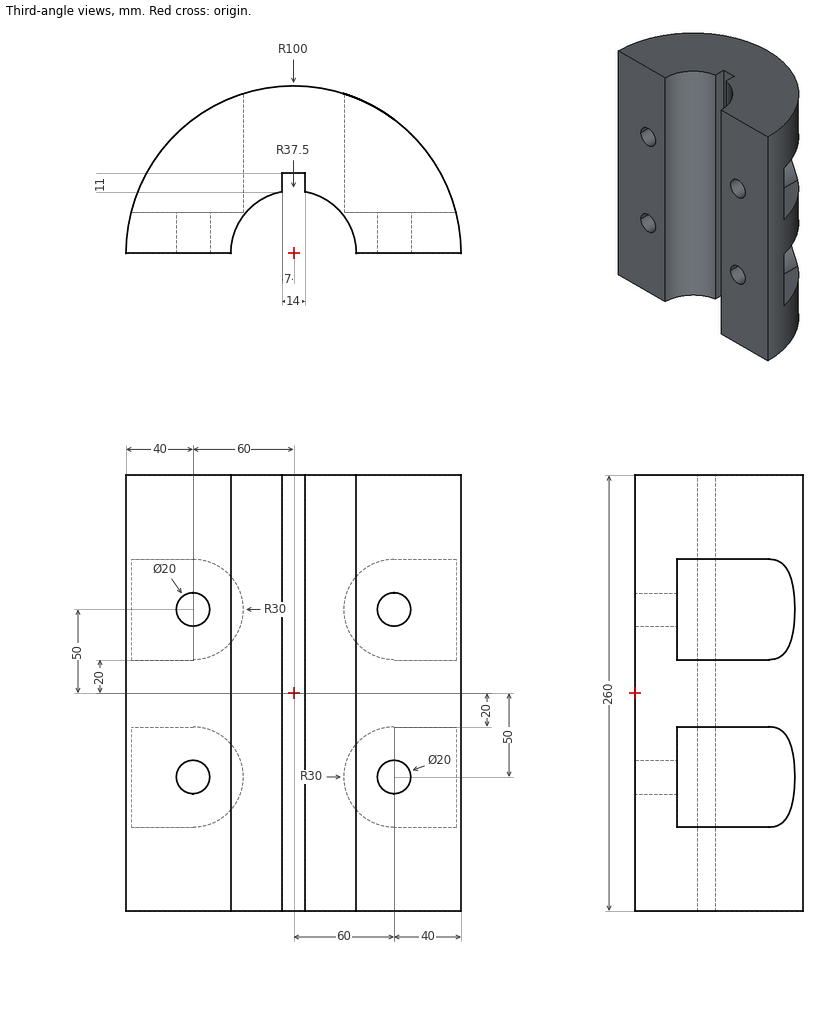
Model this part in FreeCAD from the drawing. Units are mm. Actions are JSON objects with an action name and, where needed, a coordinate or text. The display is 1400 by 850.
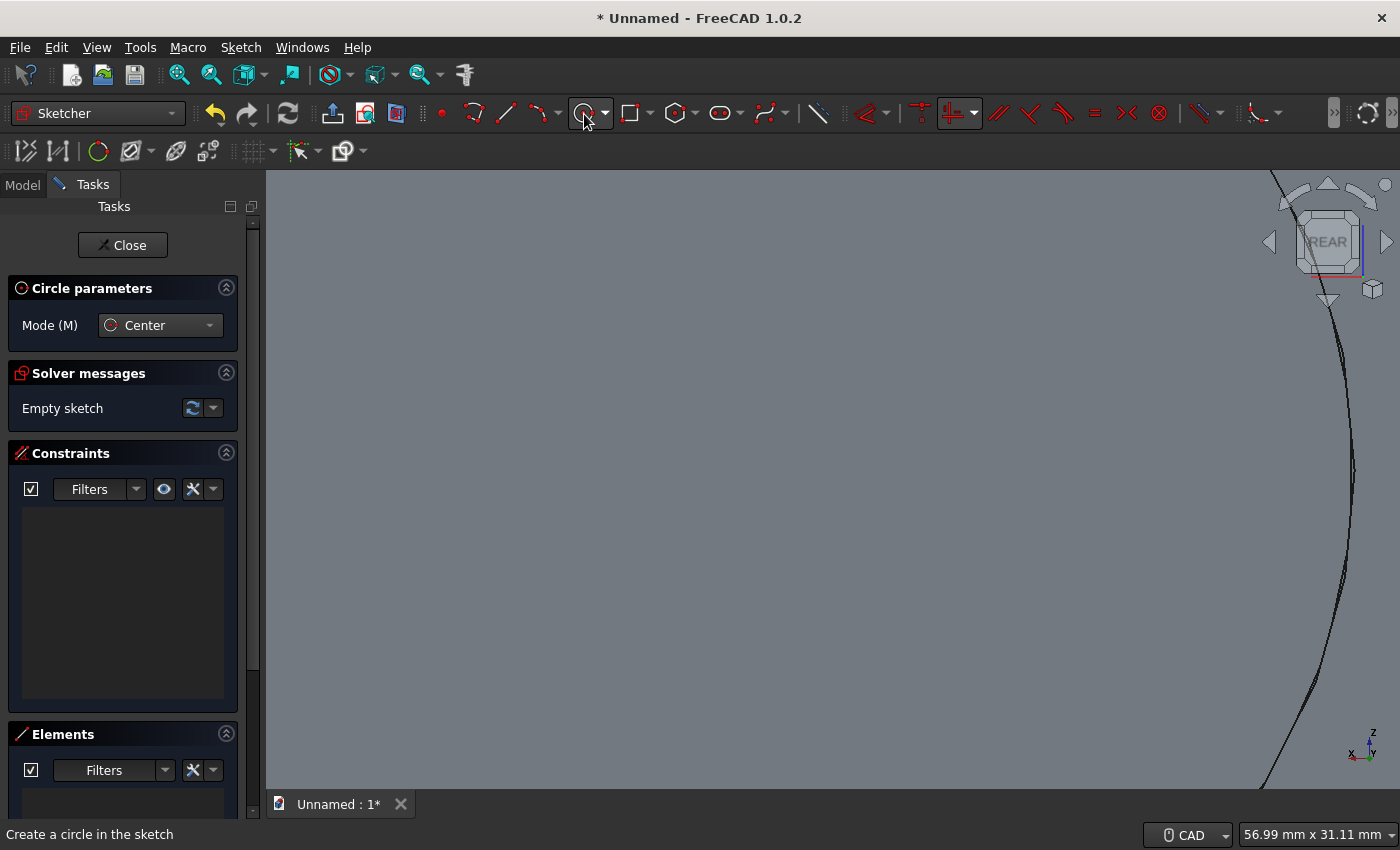
{"action": "left_click", "coordinate": [758, 470]}
{"action": "left_click", "coordinate": [898, 330]}
{"action": "key", "text": "Escape"}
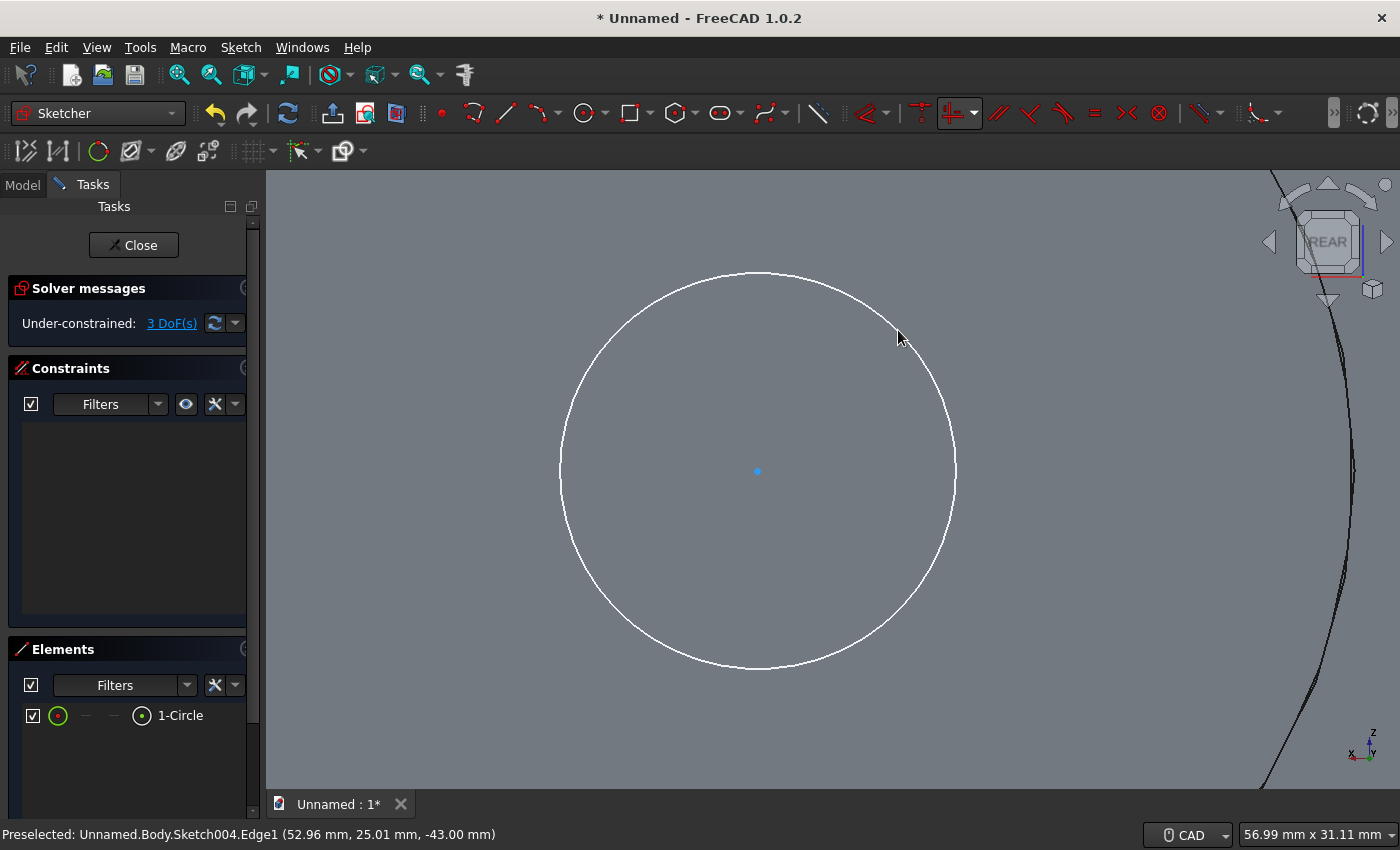
{"action": "left_click", "coordinate": [866, 114]}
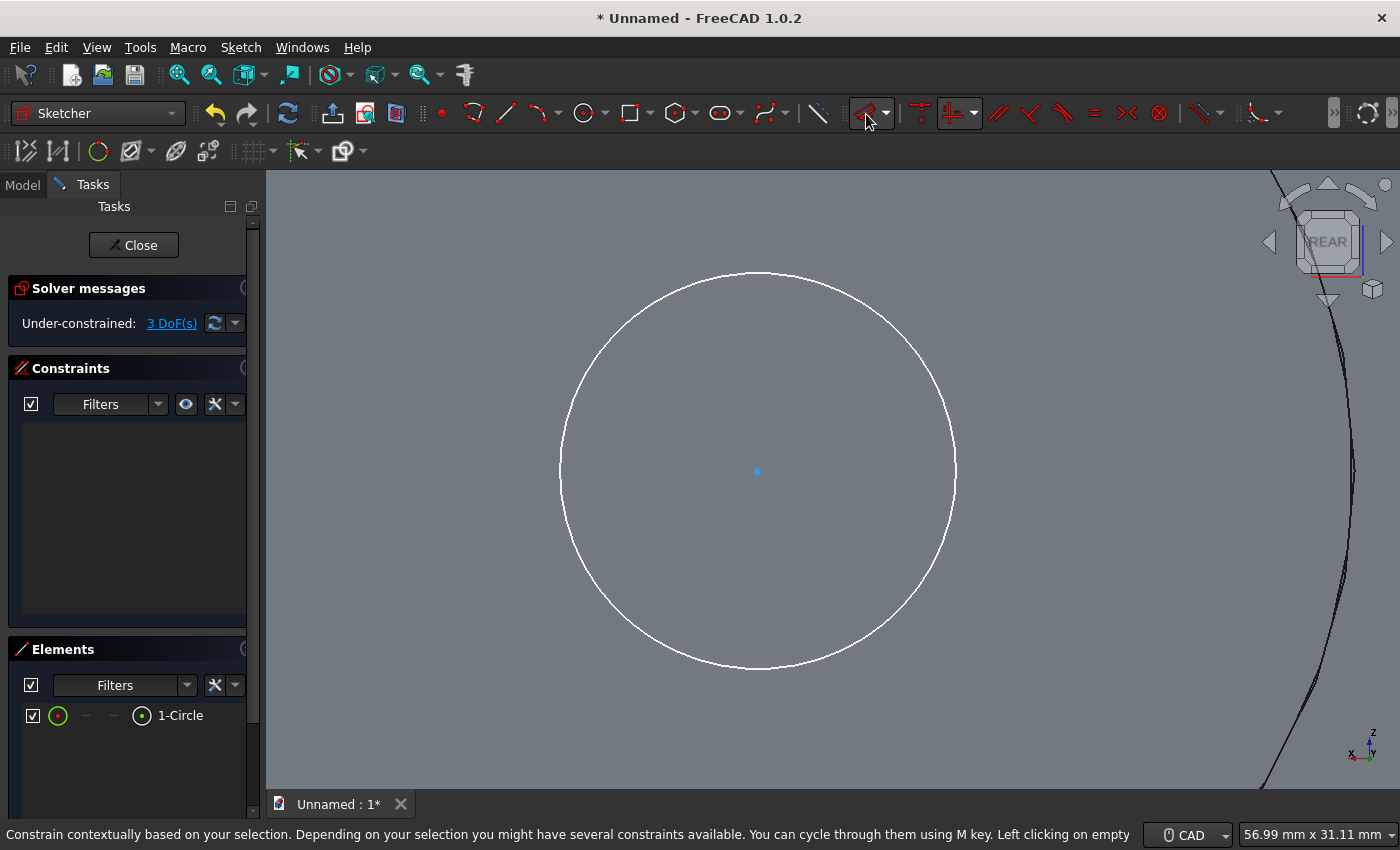
{"action": "left_click", "coordinate": [898, 331]}
{"action": "left_click", "coordinate": [921, 308]}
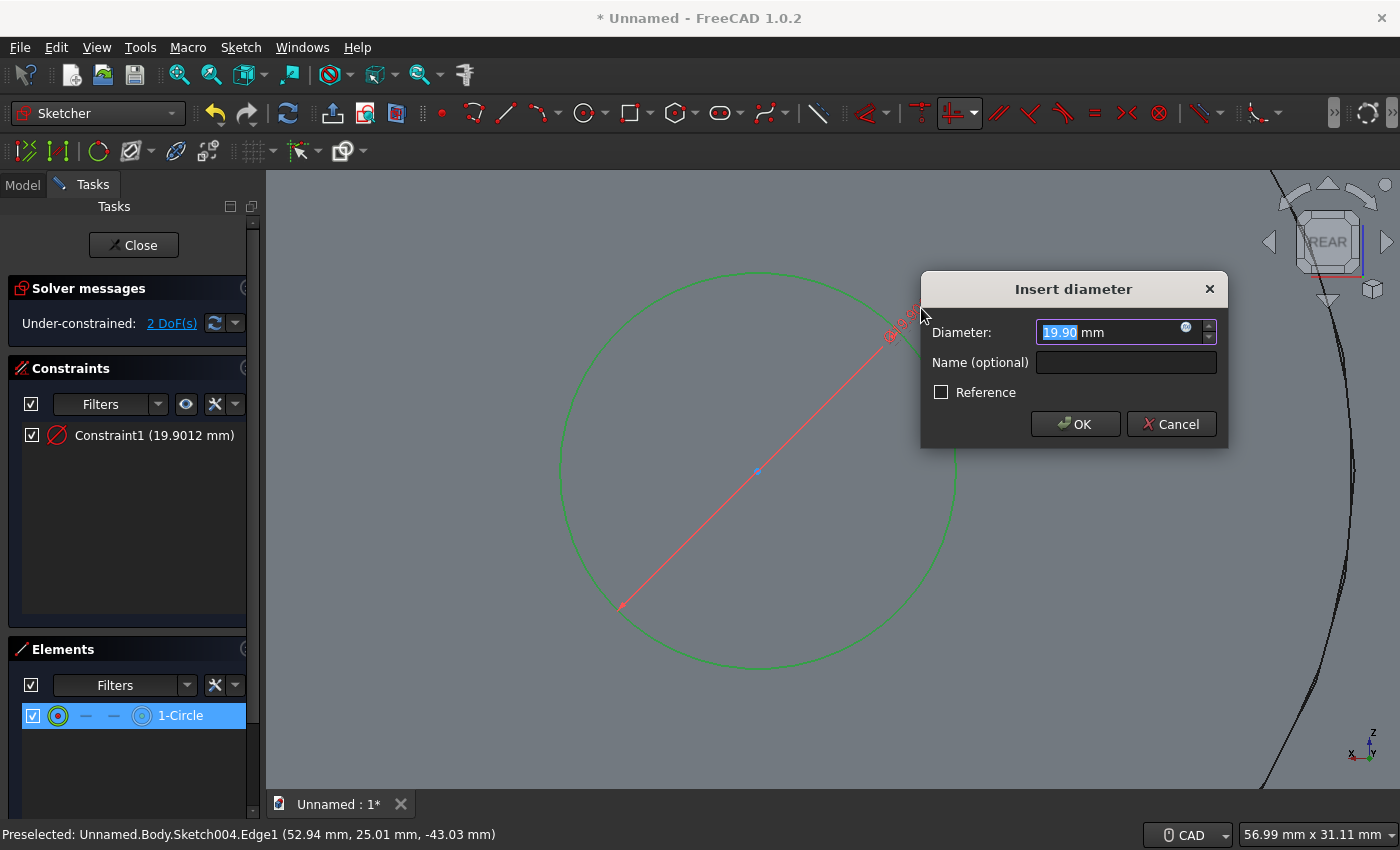
{"action": "type", "text": "20"}
{"action": "key", "text": "Return"}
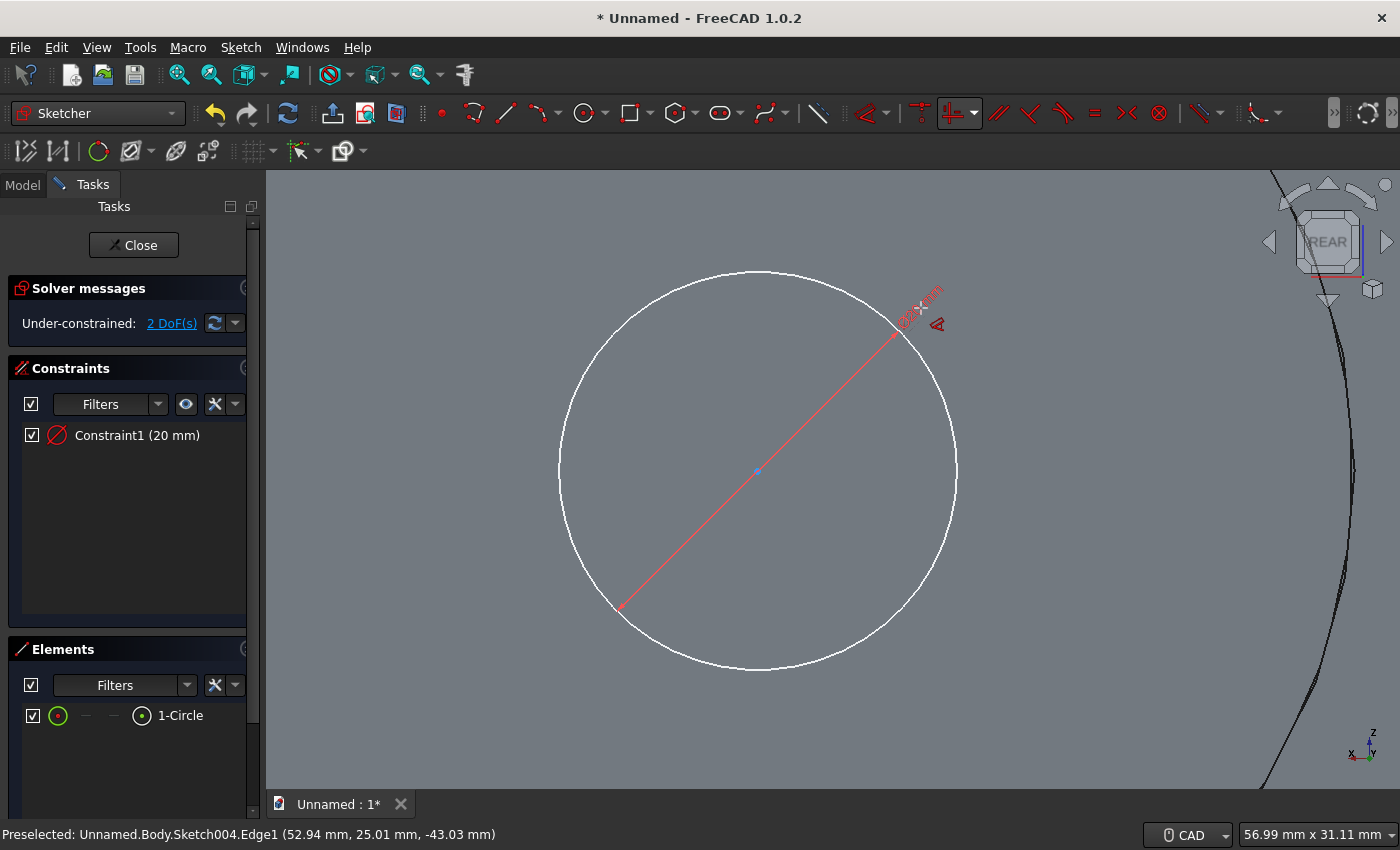
{"action": "left_click", "coordinate": [758, 471]}
{"action": "left_click", "coordinate": [997, 505]}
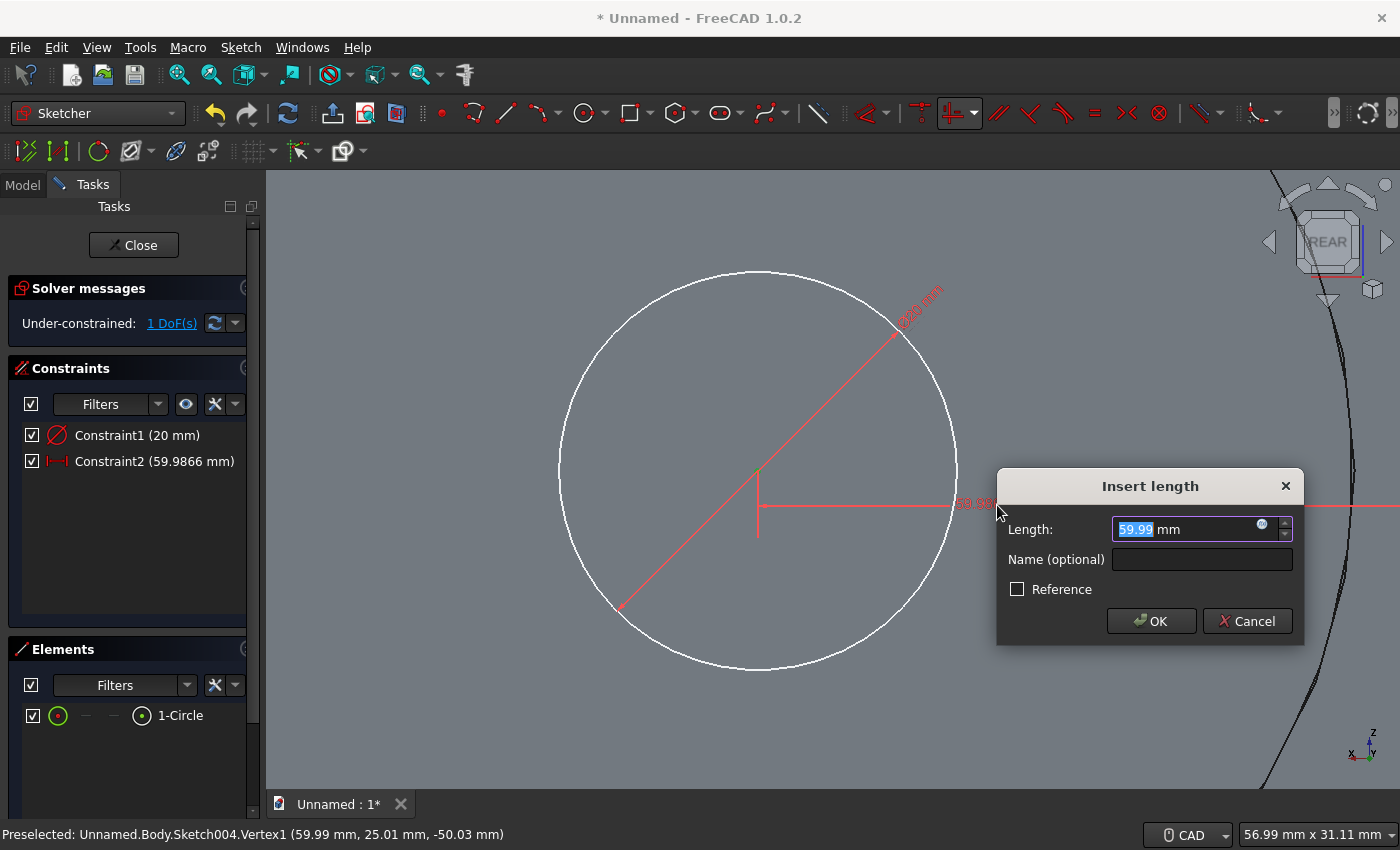
{"action": "type", "text": "60"}
{"action": "key", "text": "Return"}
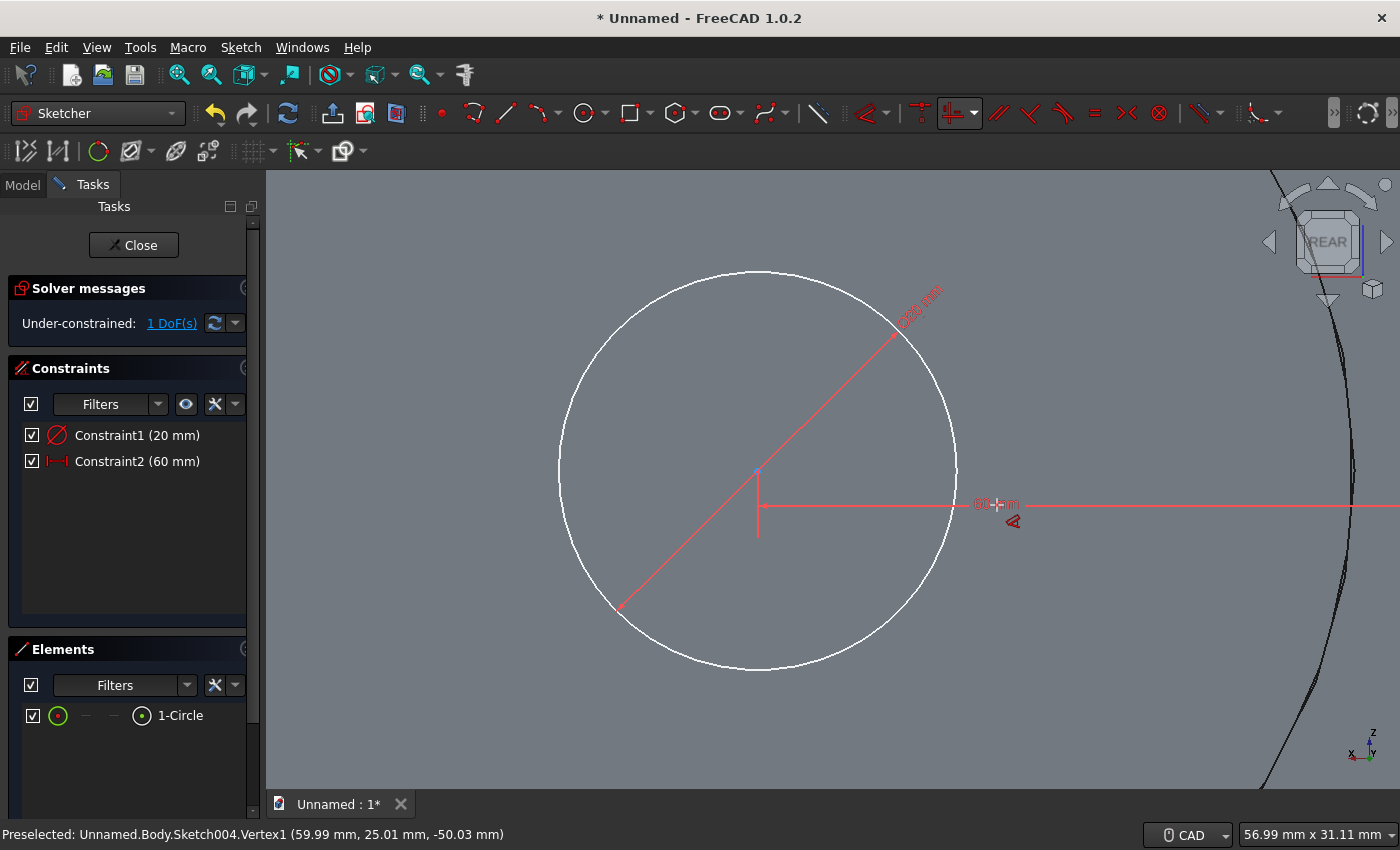
{"action": "left_click", "coordinate": [758, 471]}
{"action": "left_click", "coordinate": [724, 335]}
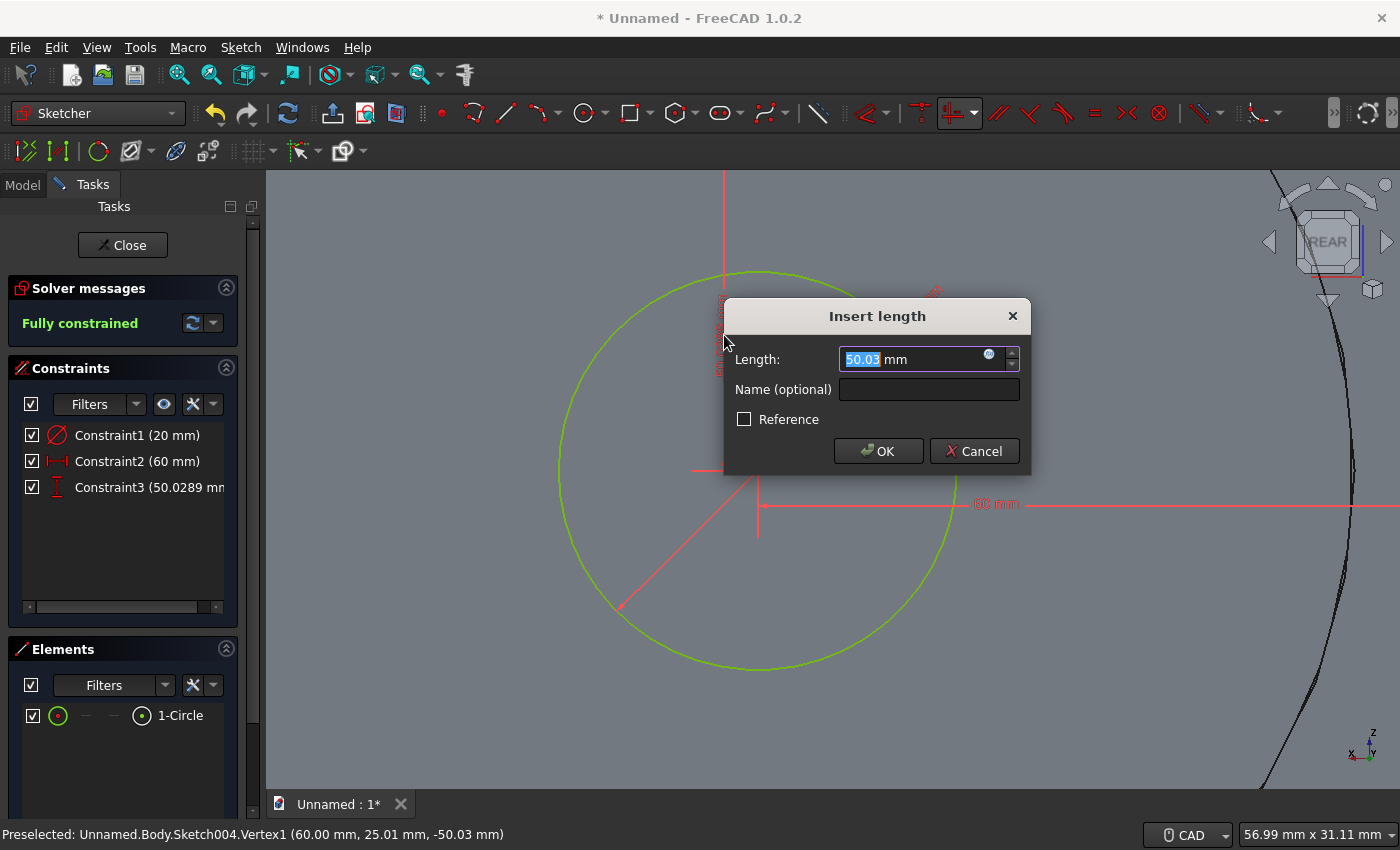
{"action": "type", "text": "50"}
{"action": "key", "text": "Return"}
{"action": "key", "text": "Escape"}